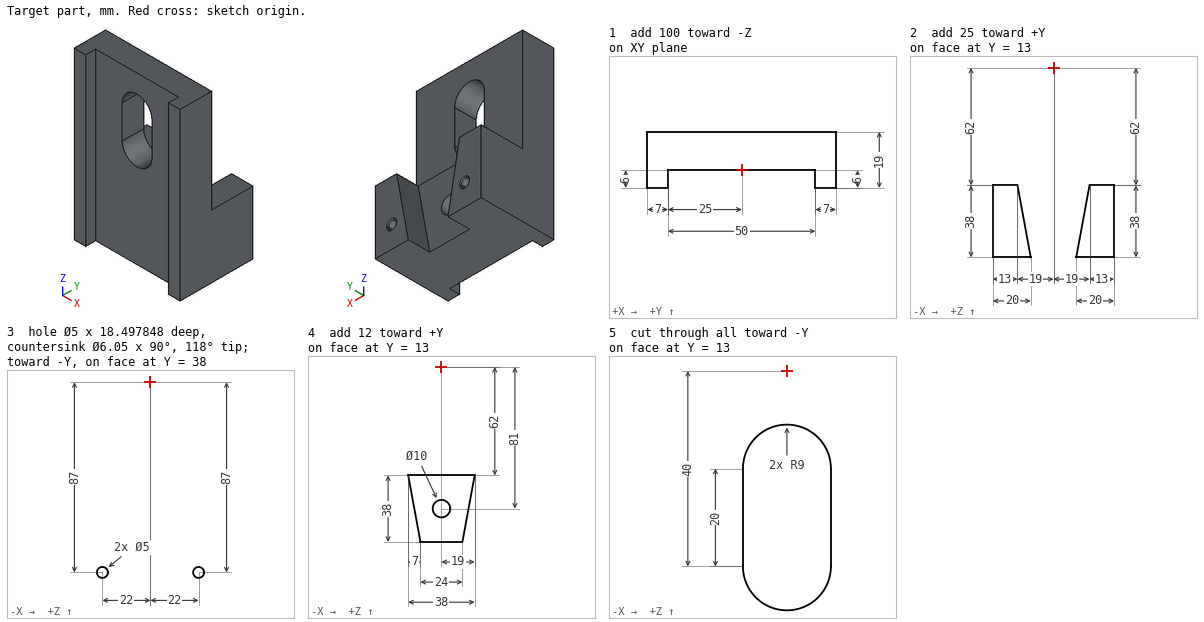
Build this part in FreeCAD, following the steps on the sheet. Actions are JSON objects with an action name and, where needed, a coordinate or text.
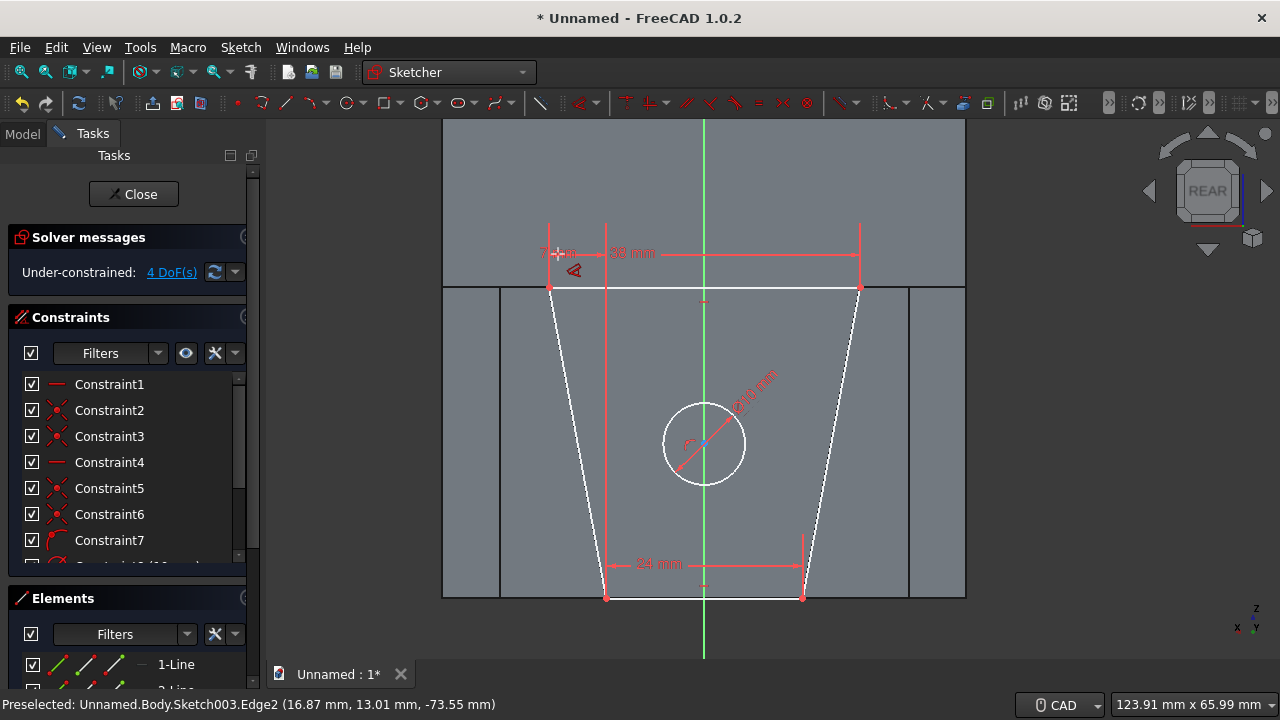
{"action": "left_click", "coordinate": [704, 444]}
{"action": "left_click", "coordinate": [738, 227]}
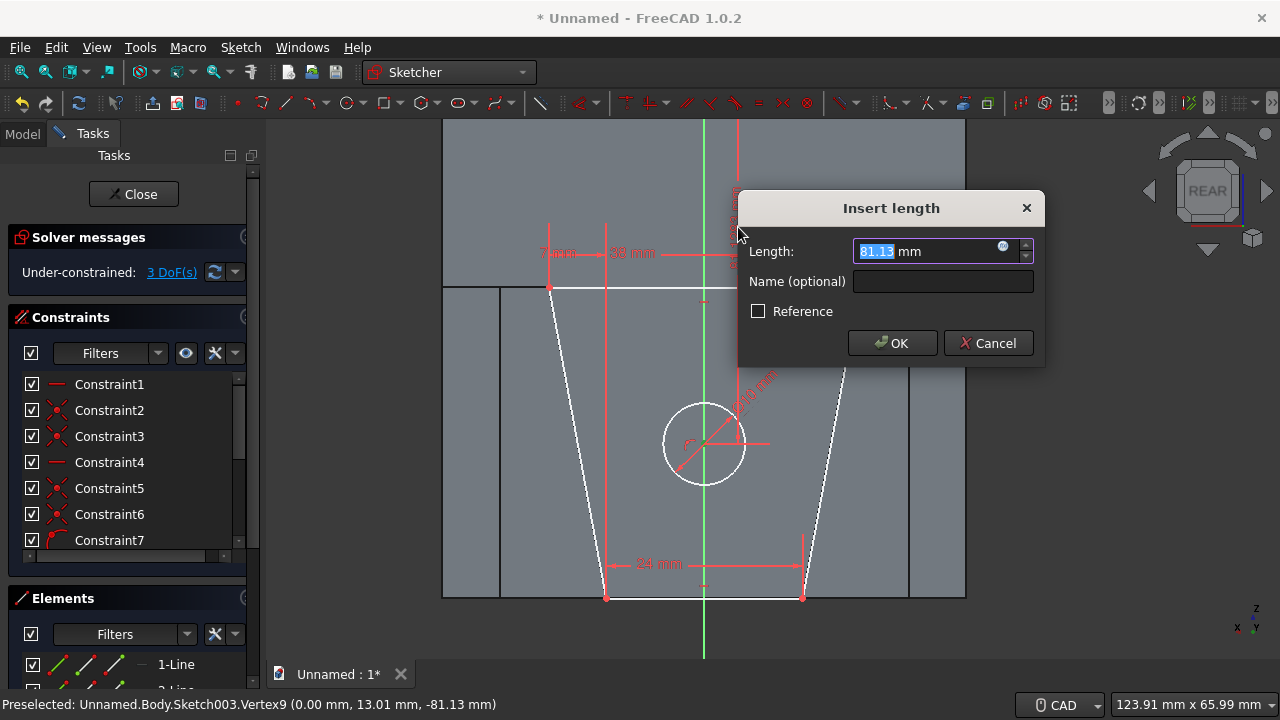
{"action": "type", "text": "81"}
{"action": "key", "text": "Return"}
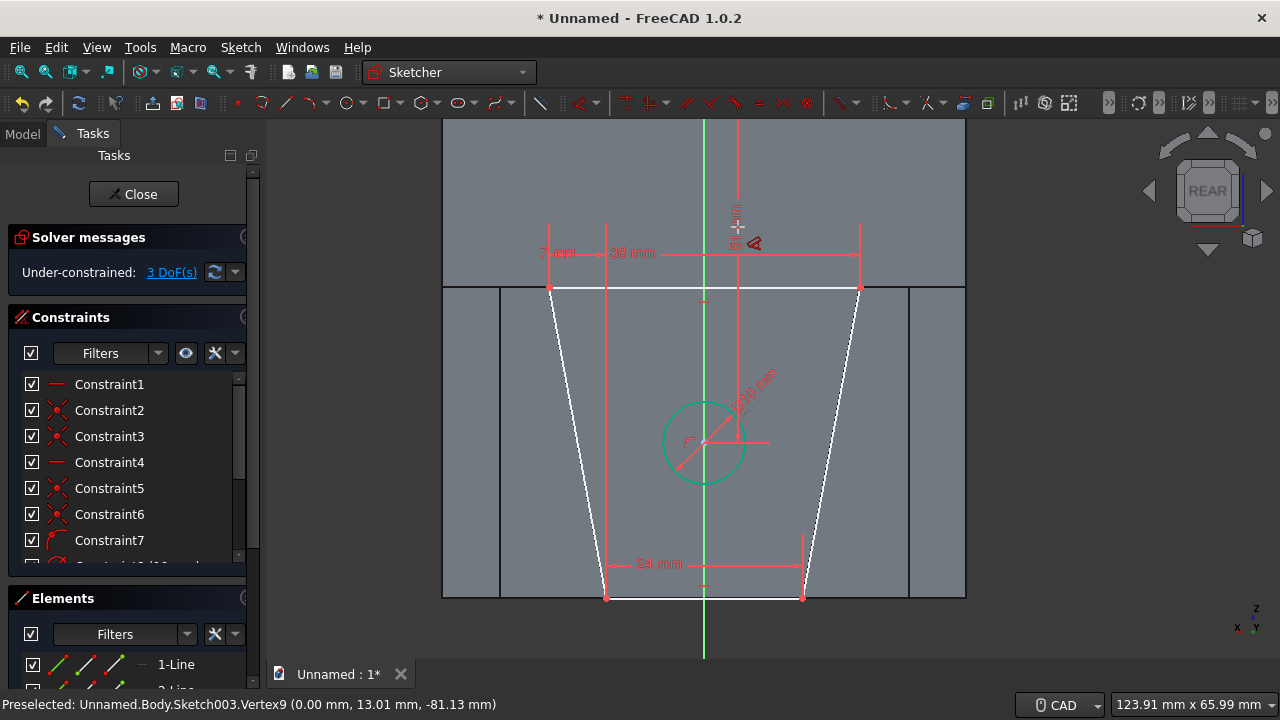
{"action": "left_click", "coordinate": [860, 288]}
{"action": "left_click", "coordinate": [782, 322]}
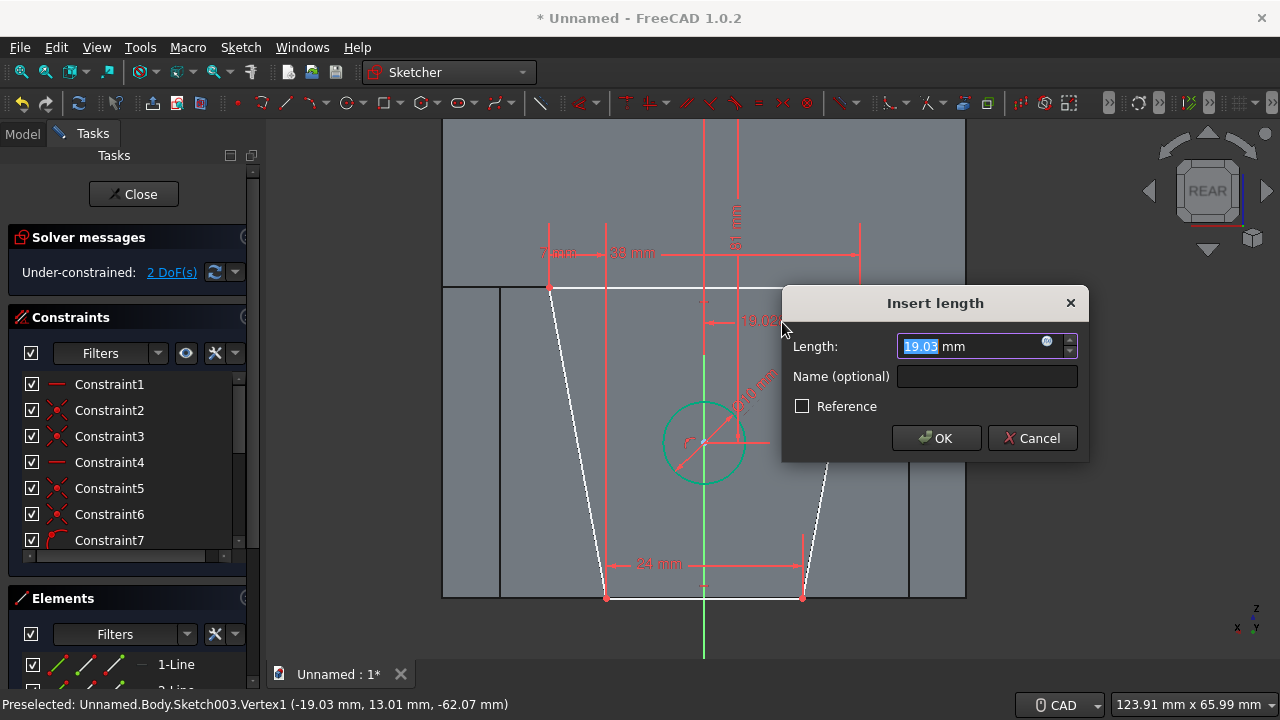
{"action": "type", "text": "19"}
{"action": "key", "text": "Return"}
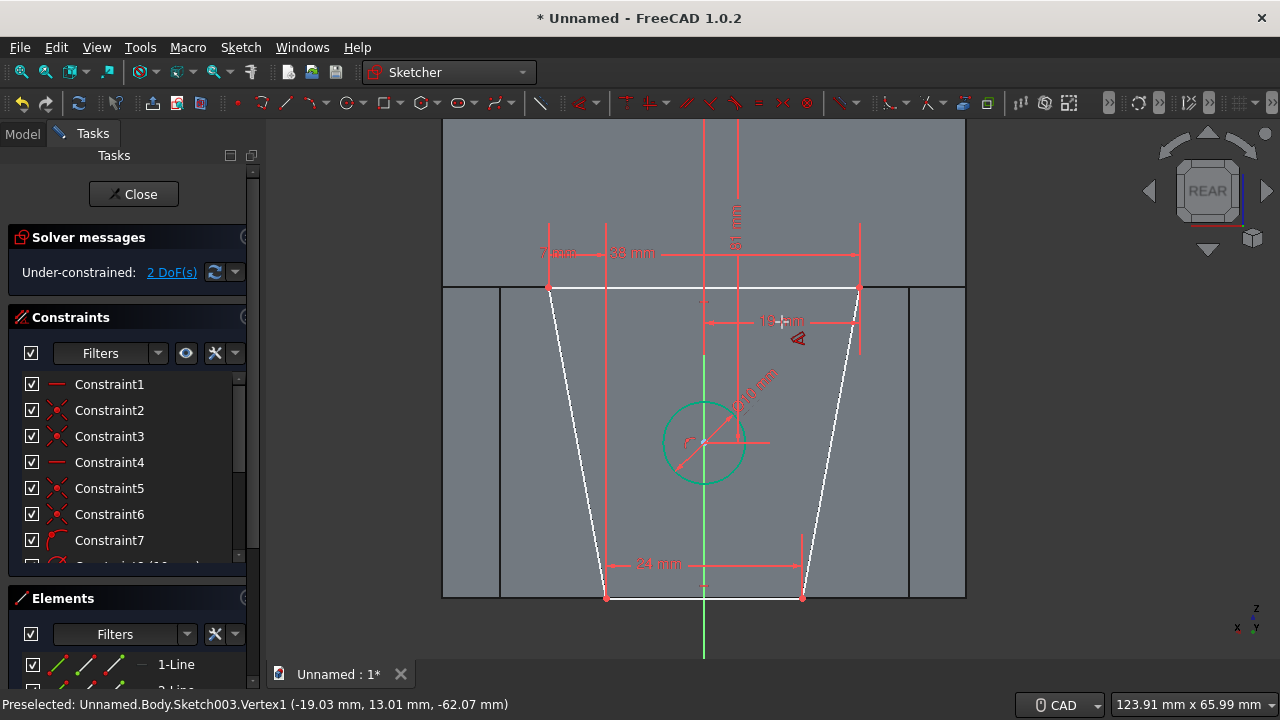
{"action": "left_click", "coordinate": [860, 288]}
{"action": "left_click", "coordinate": [894, 217]}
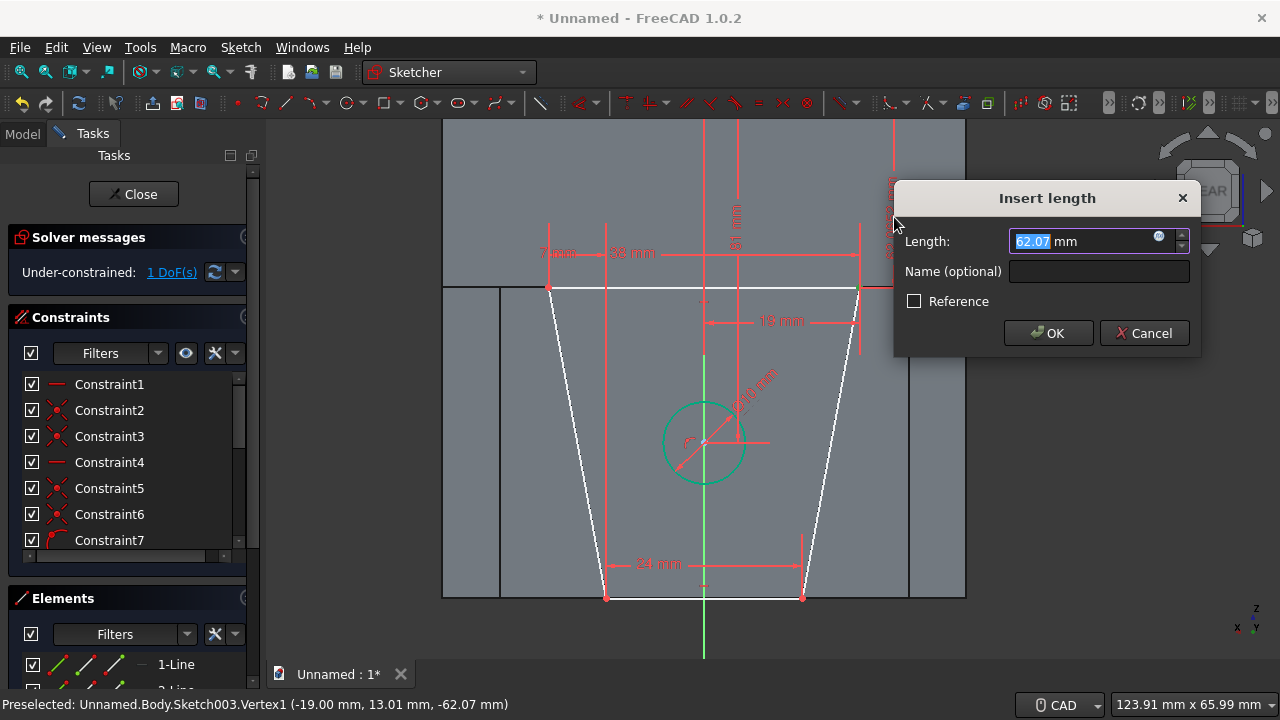
{"action": "type", "text": "62"}
{"action": "key", "text": "Return"}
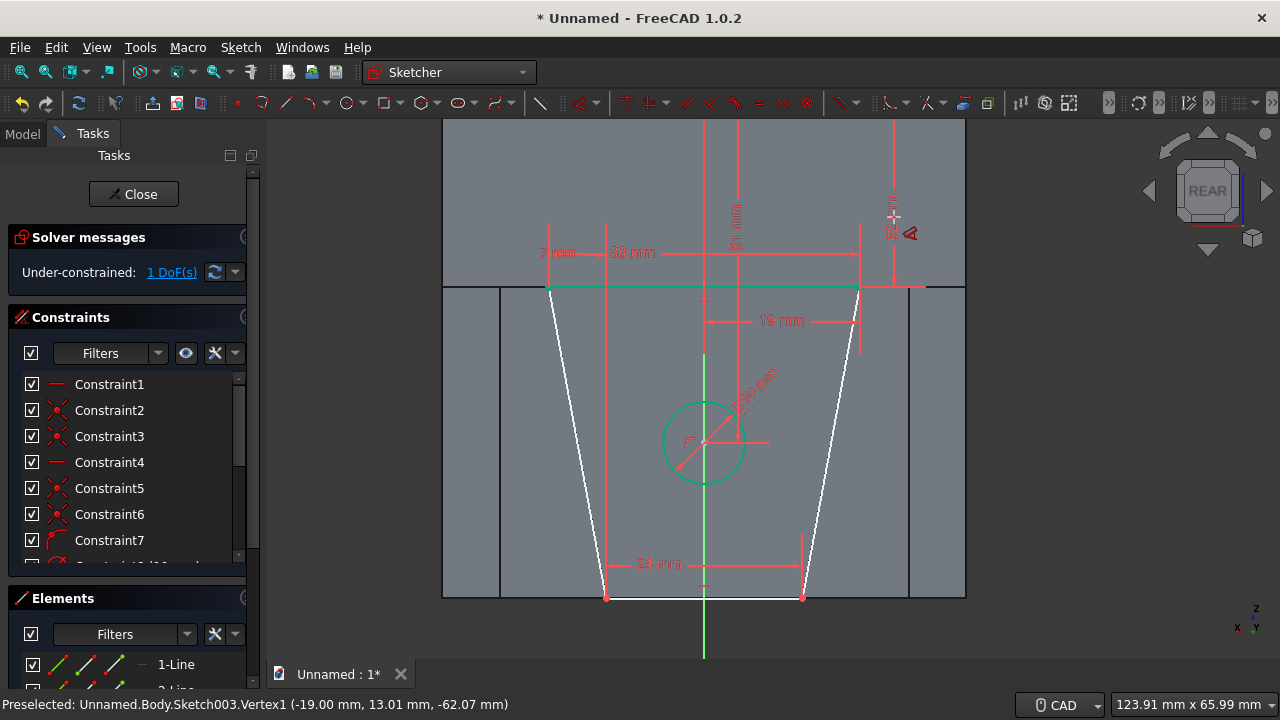
{"action": "left_click", "coordinate": [566, 381]}
{"action": "left_click", "coordinate": [515, 443]}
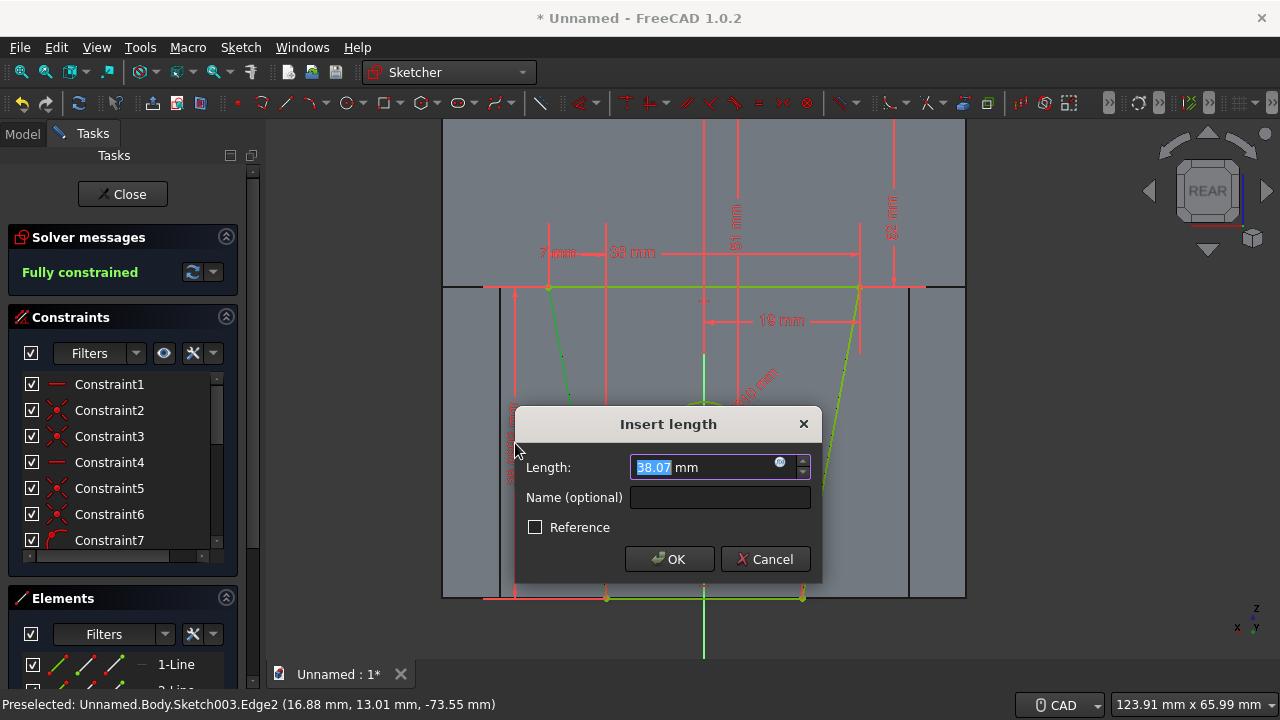
{"action": "type", "text": "38"}
{"action": "key", "text": "Return"}
{"action": "key", "text": "Escape"}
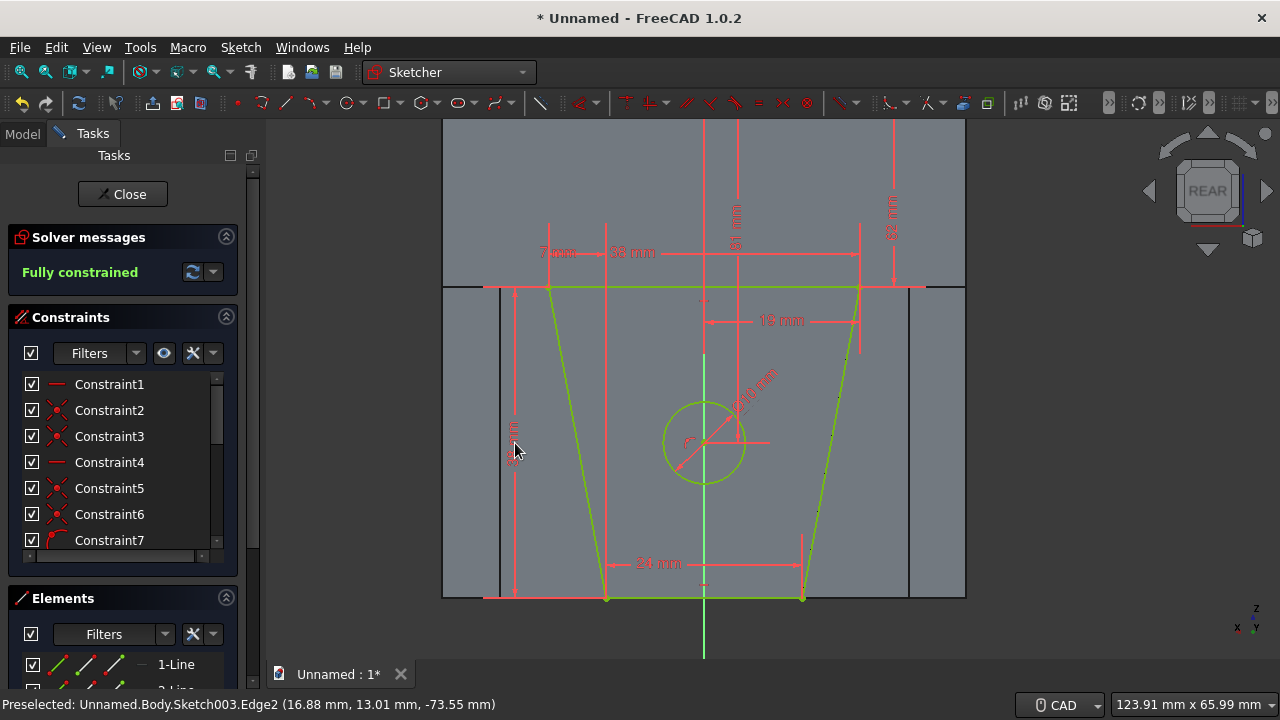
{"action": "left_click", "coordinate": [123, 194]}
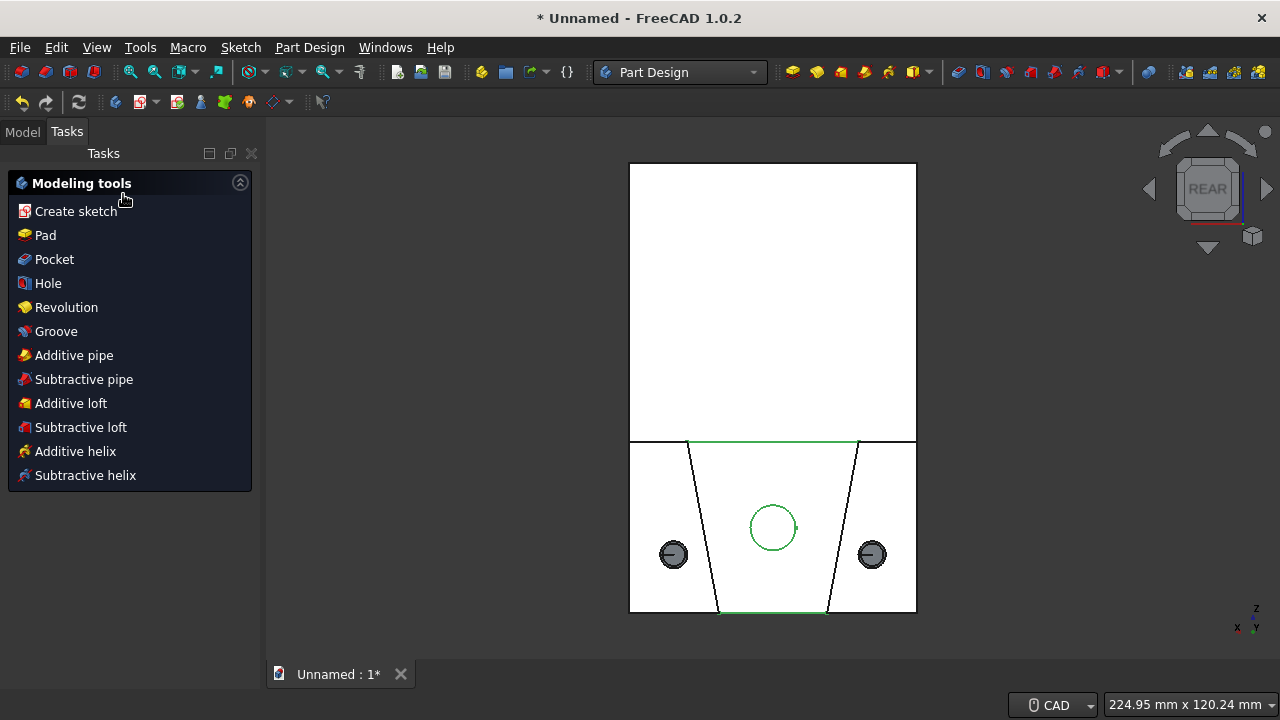
{"action": "left_click", "coordinate": [794, 72]}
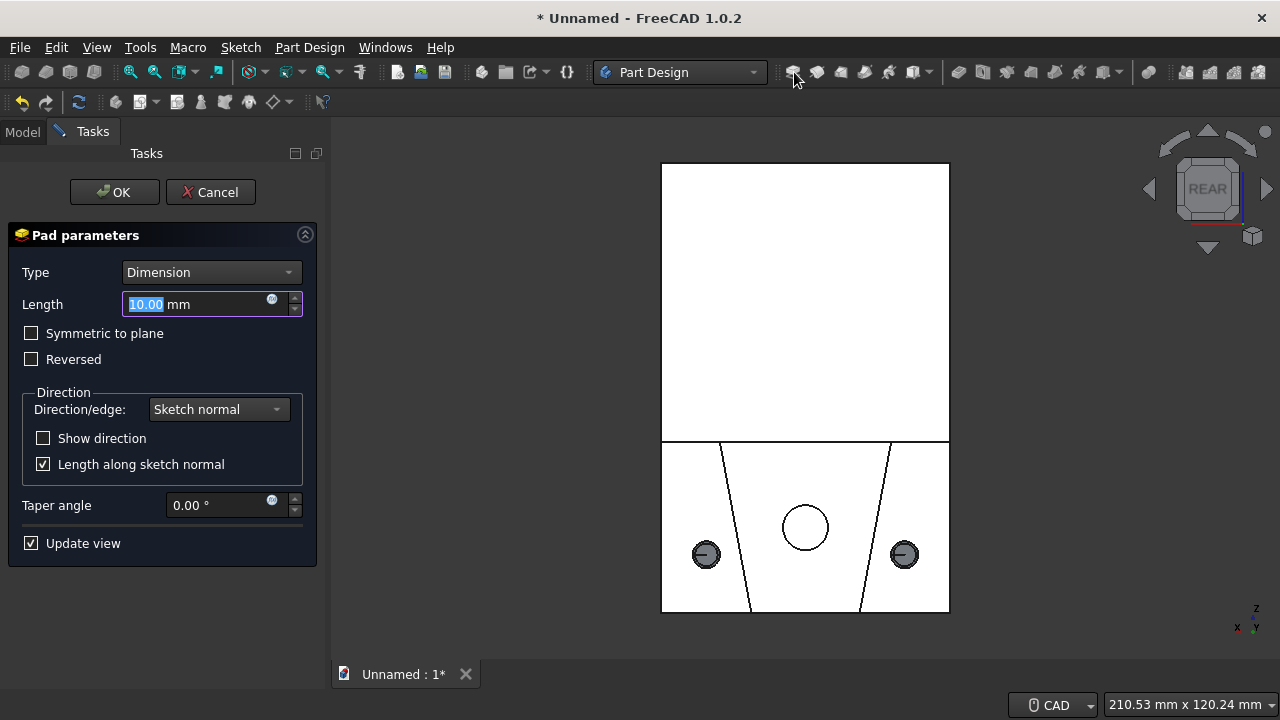
{"action": "type", "text": "12"}
{"action": "key", "text": "Tab"}